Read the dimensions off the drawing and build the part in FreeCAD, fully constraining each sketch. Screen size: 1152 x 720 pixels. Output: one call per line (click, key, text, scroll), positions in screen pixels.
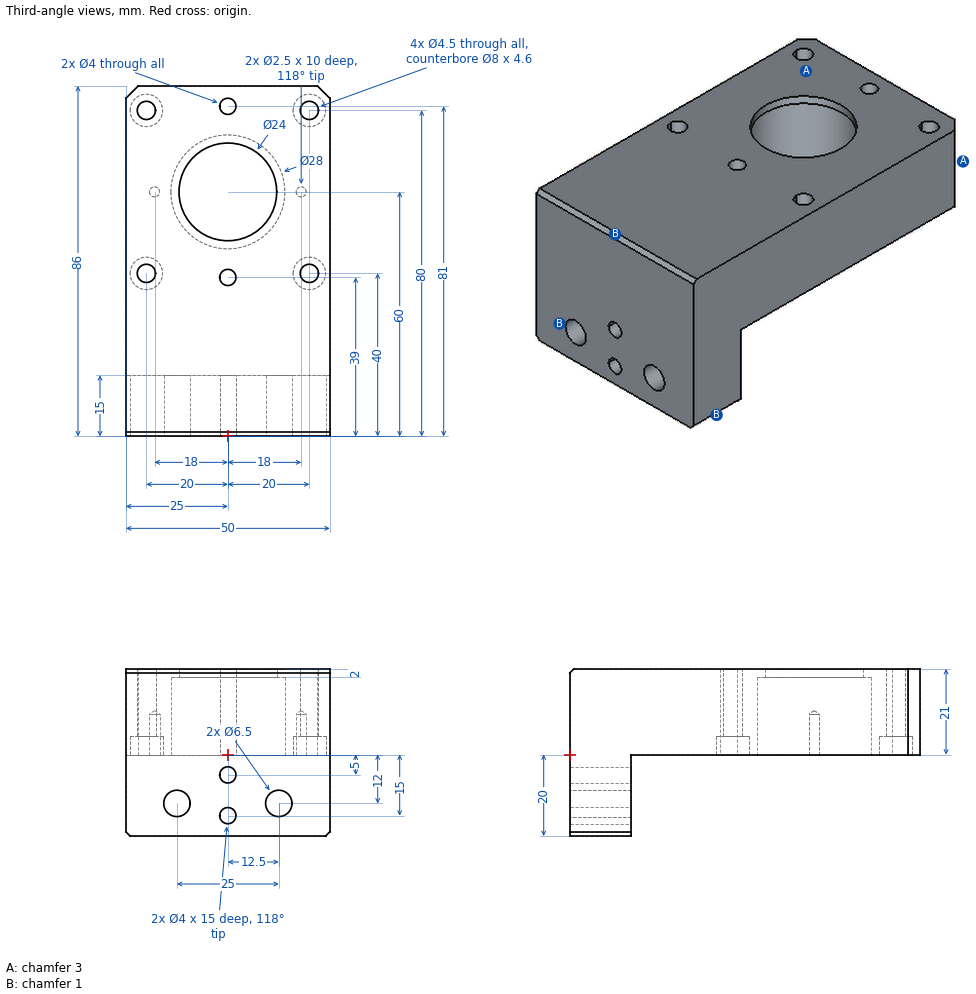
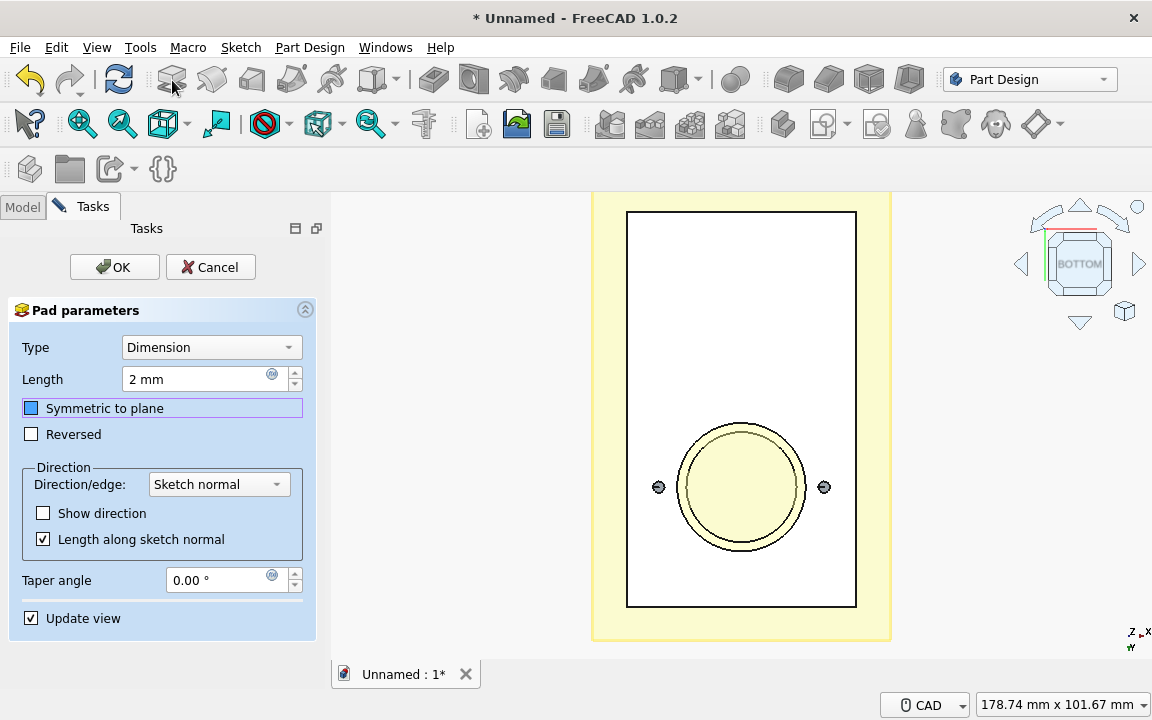
click(115, 267)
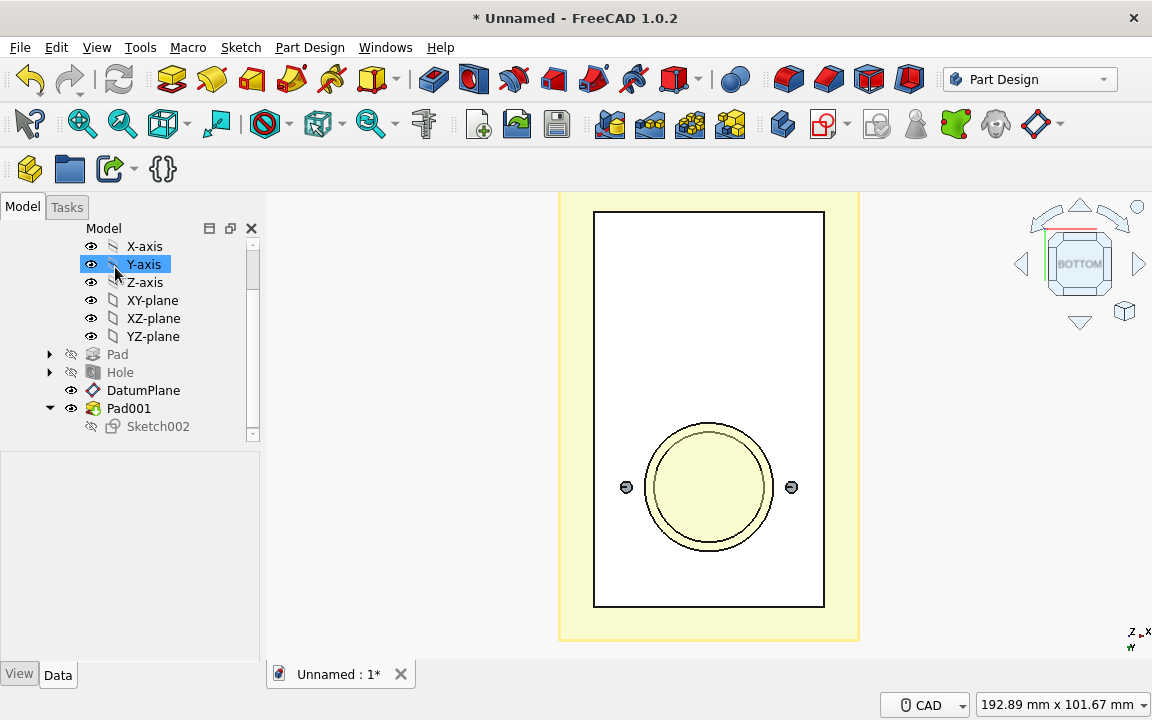
click(116, 390)
key(space)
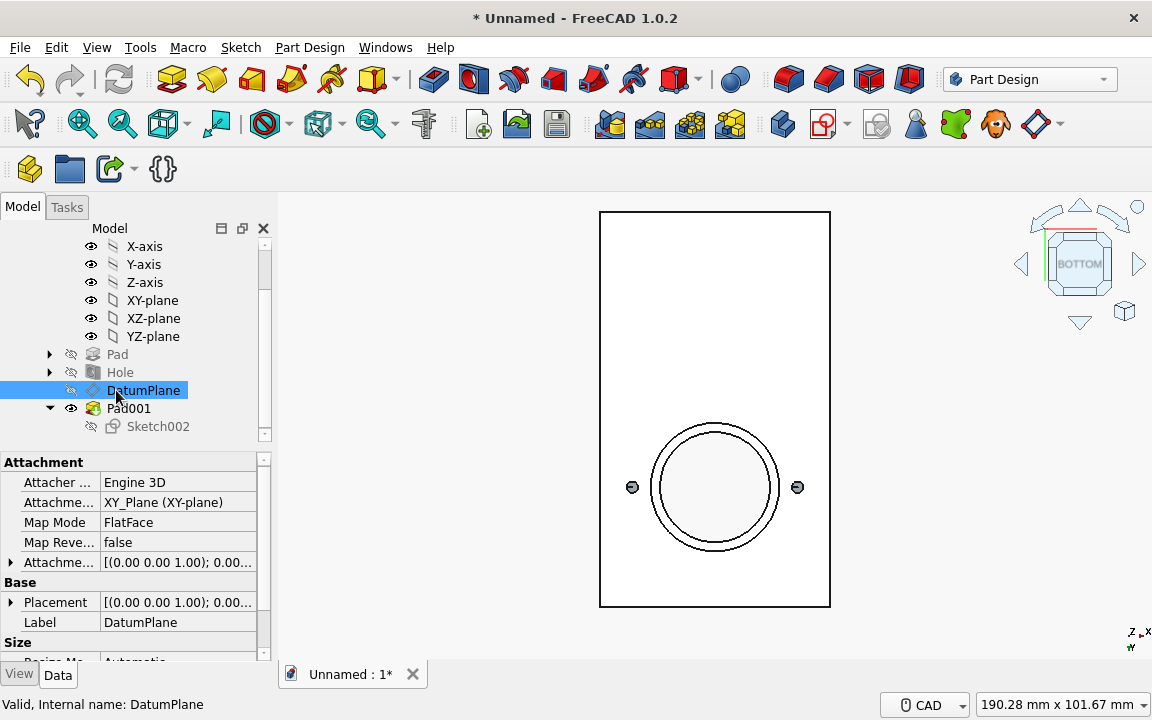
key(0)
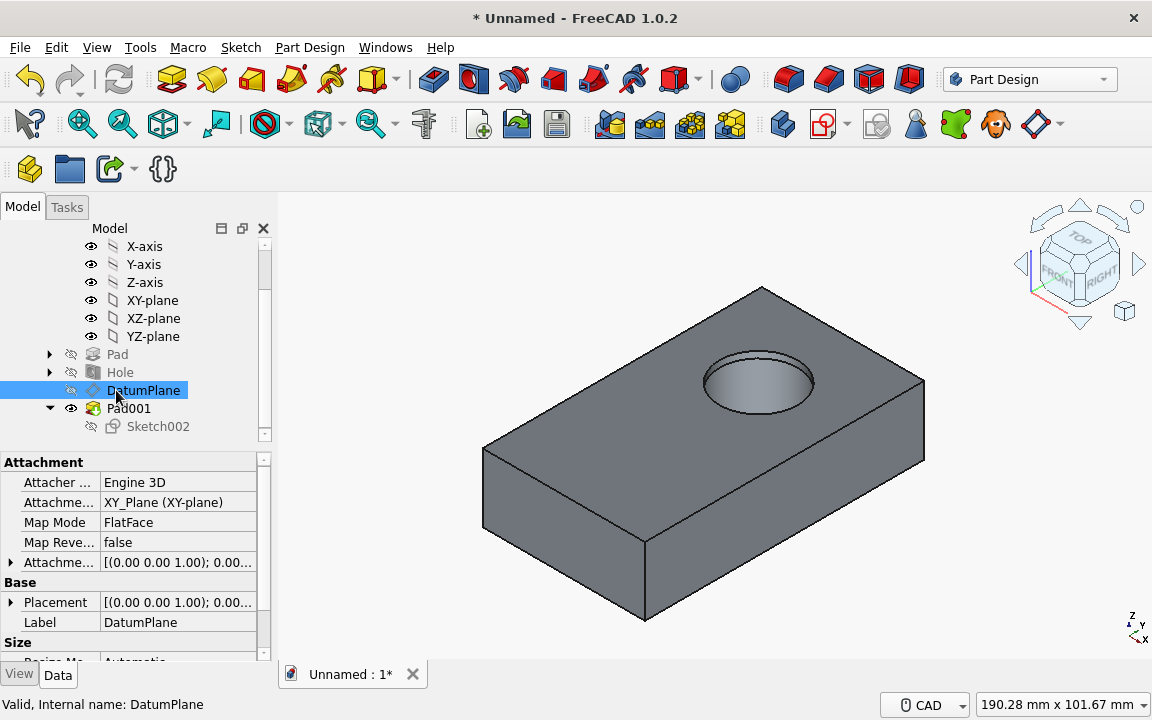
click(624, 460)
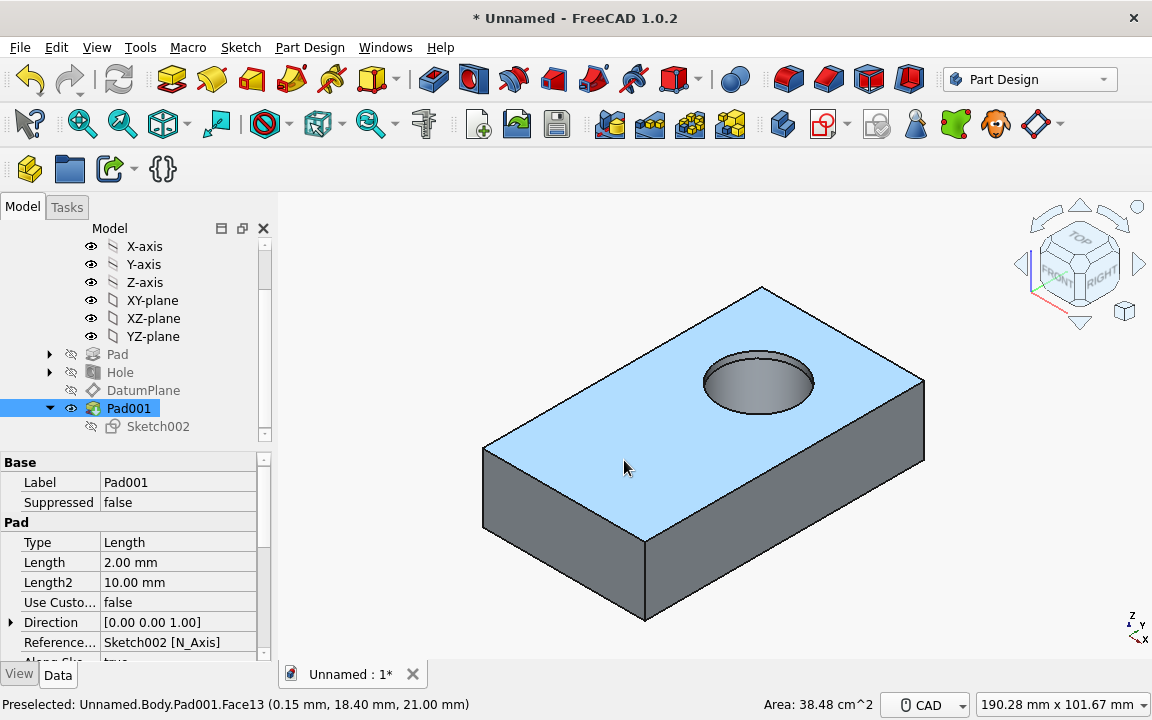
click(824, 124)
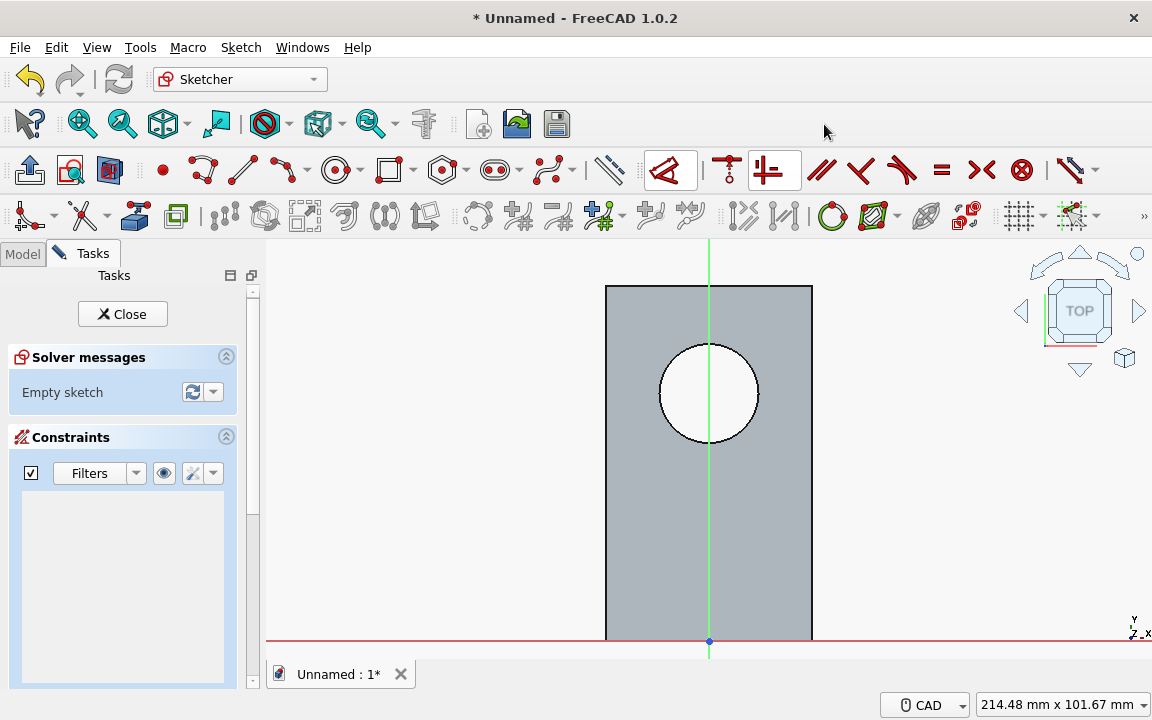
scroll(331, 354, down, 1)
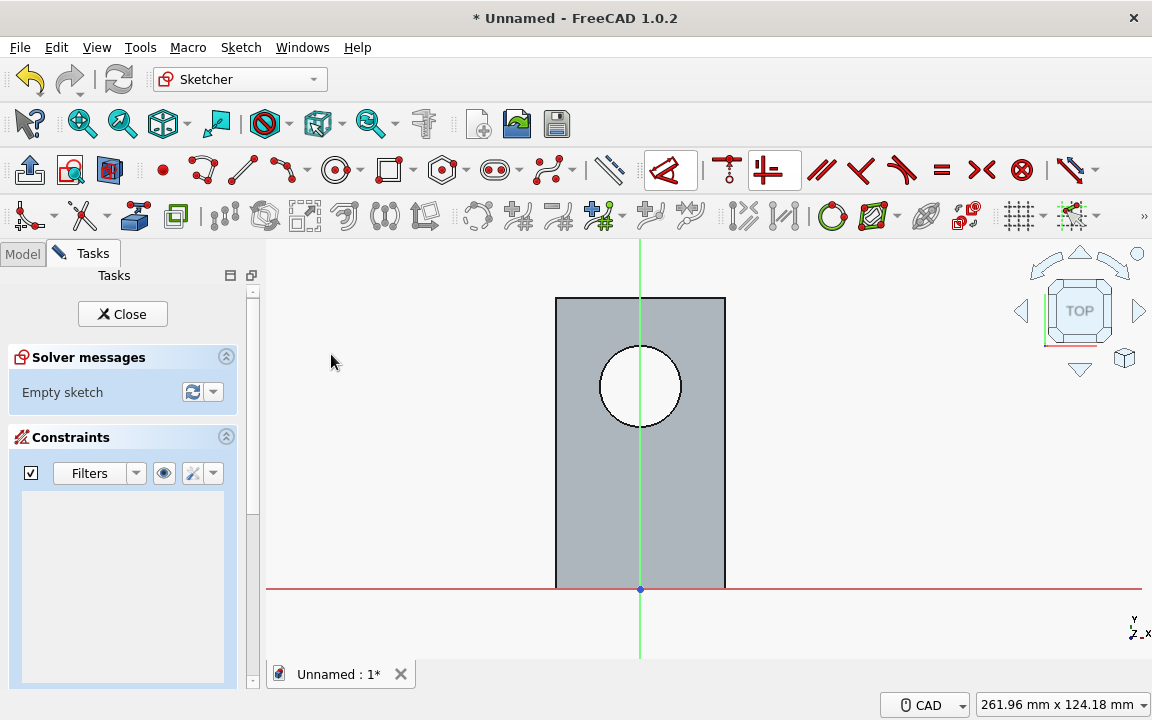
click(336, 170)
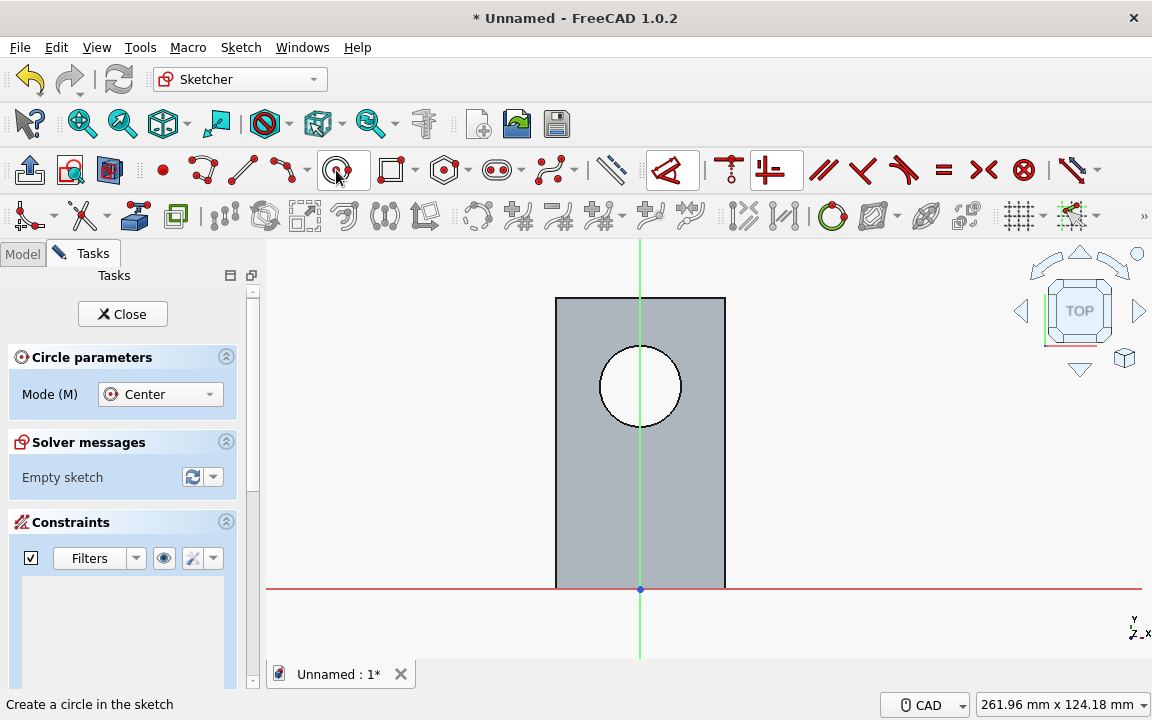
scroll(640, 315, up, 7)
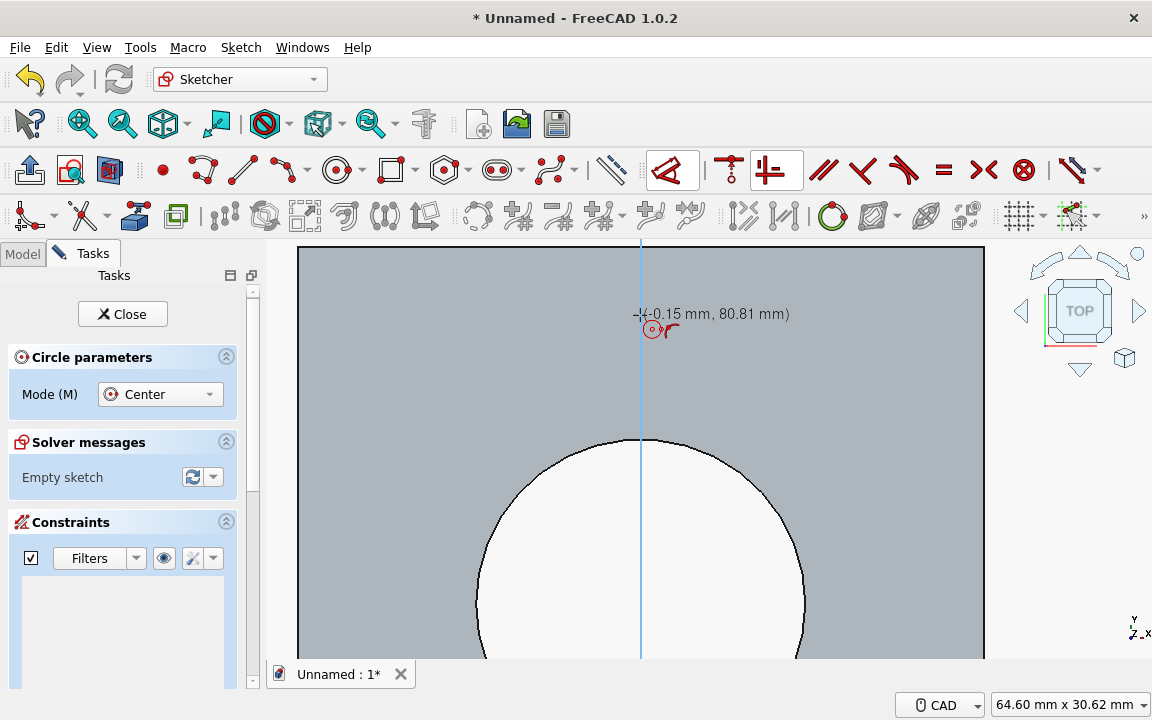
scroll(640, 315, down, 7)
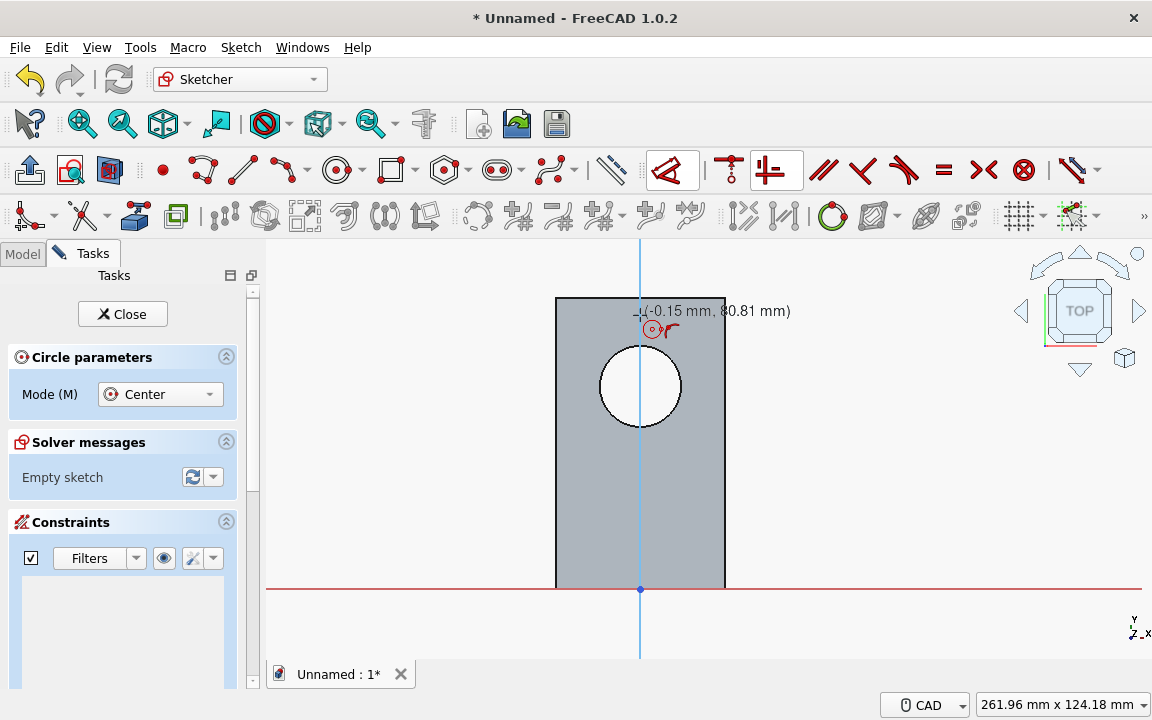
click(640, 315)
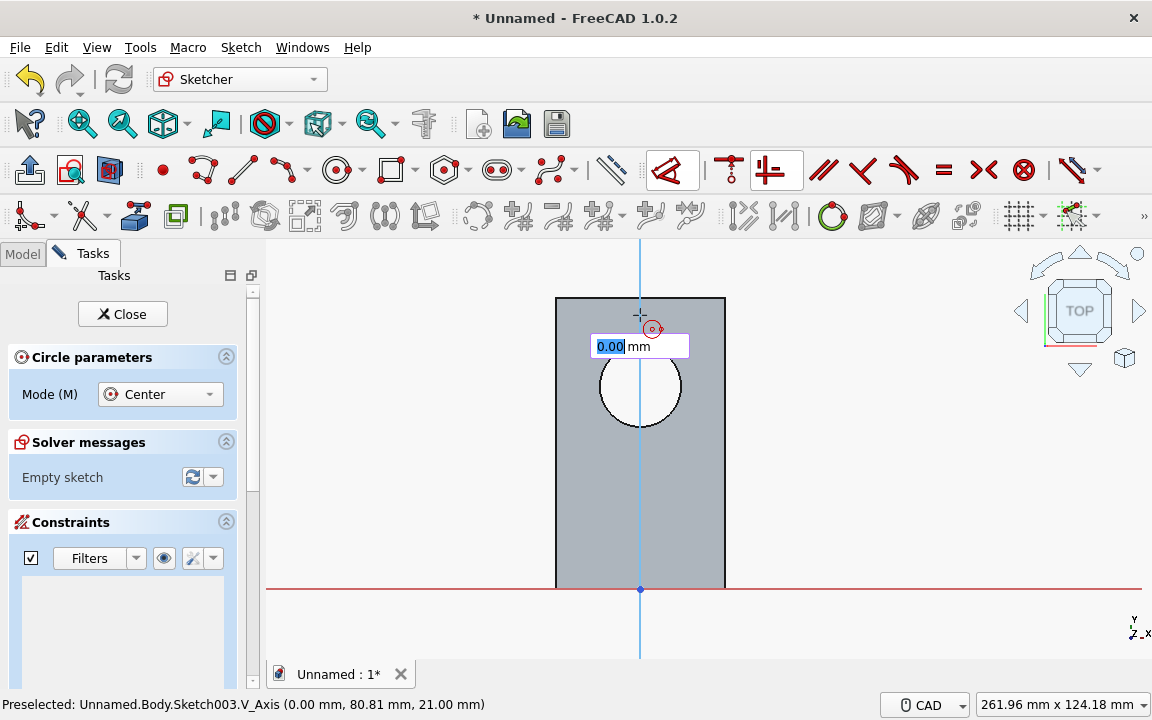
scroll(647, 313, up, 5)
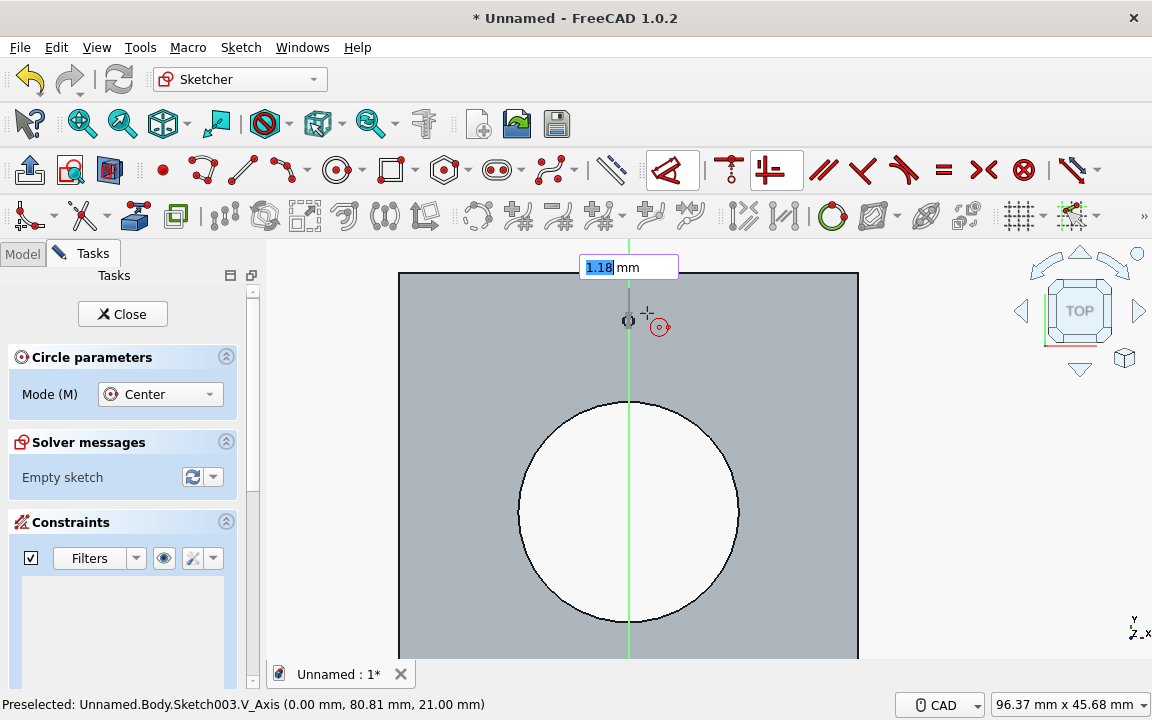
click(646, 313)